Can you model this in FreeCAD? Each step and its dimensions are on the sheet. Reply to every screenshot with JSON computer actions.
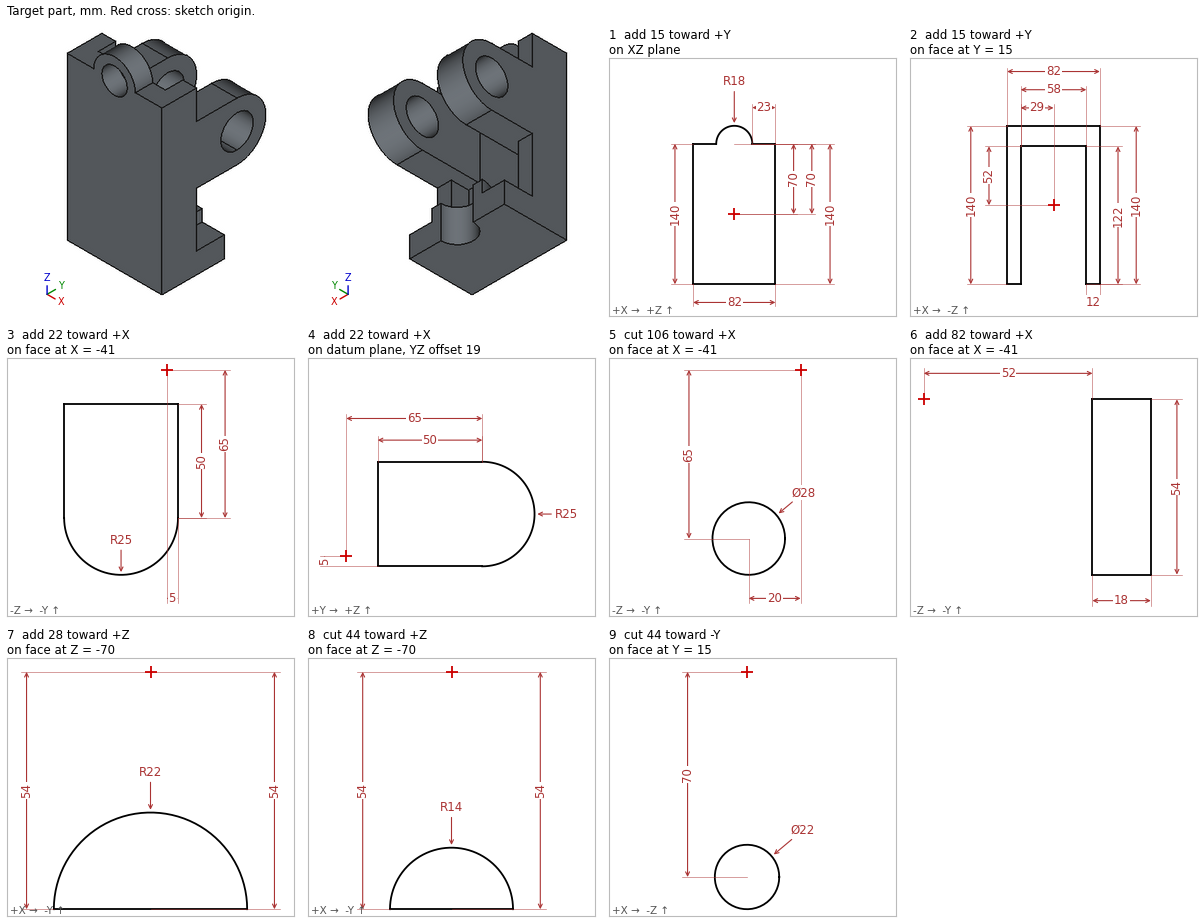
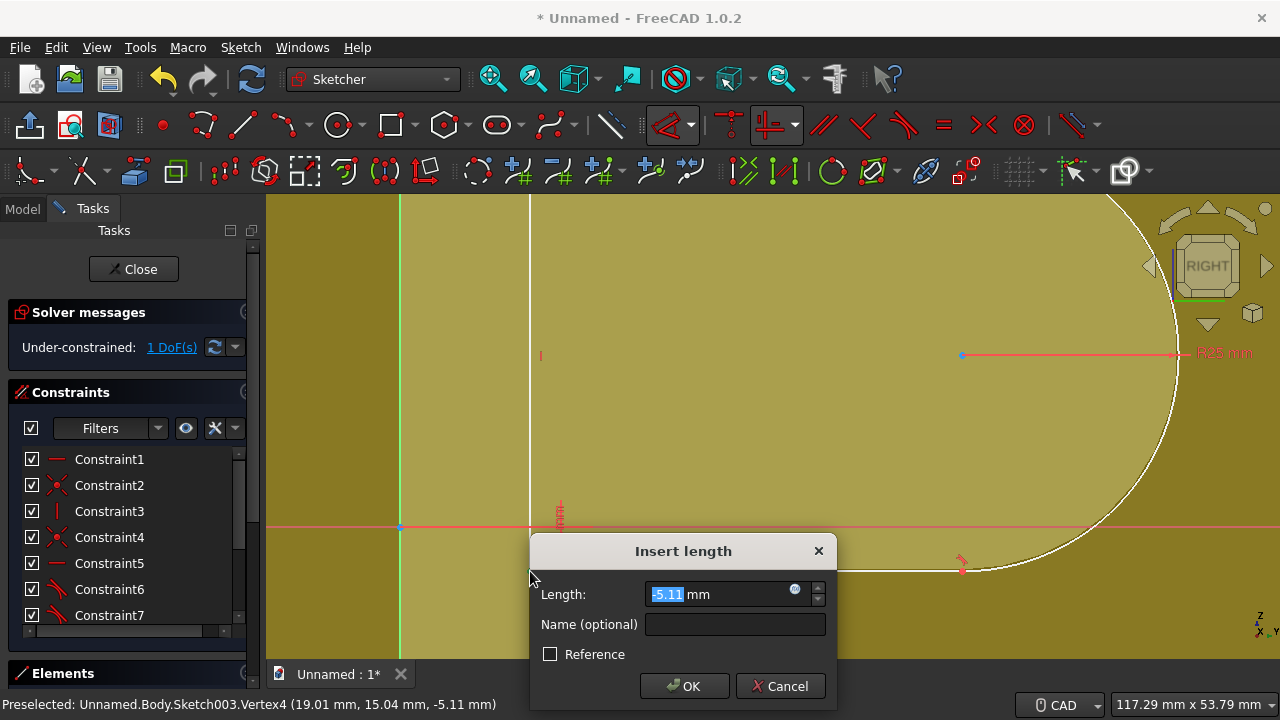
{"action": "type", "text": "-5"}
{"action": "key", "text": "Return"}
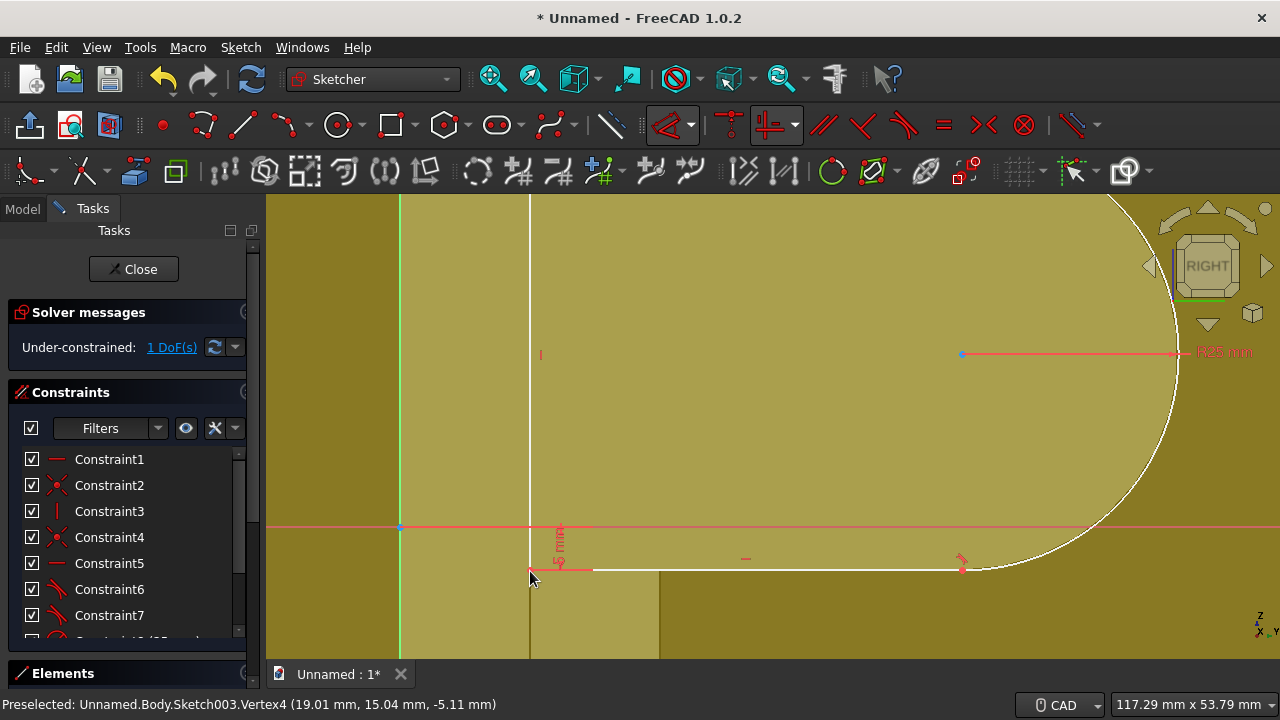
{"action": "scroll", "coordinate": [532, 573], "scroll_direction": "down", "scroll_amount": 2}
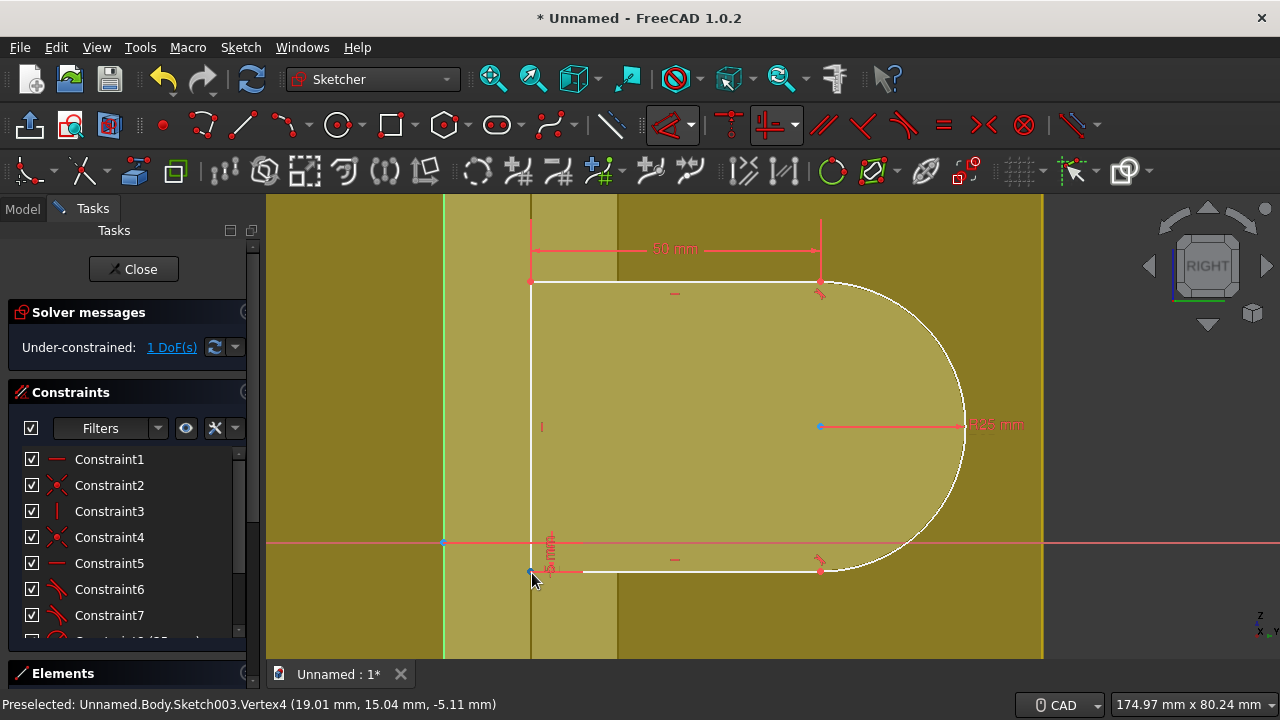
{"action": "left_click", "coordinate": [821, 282]}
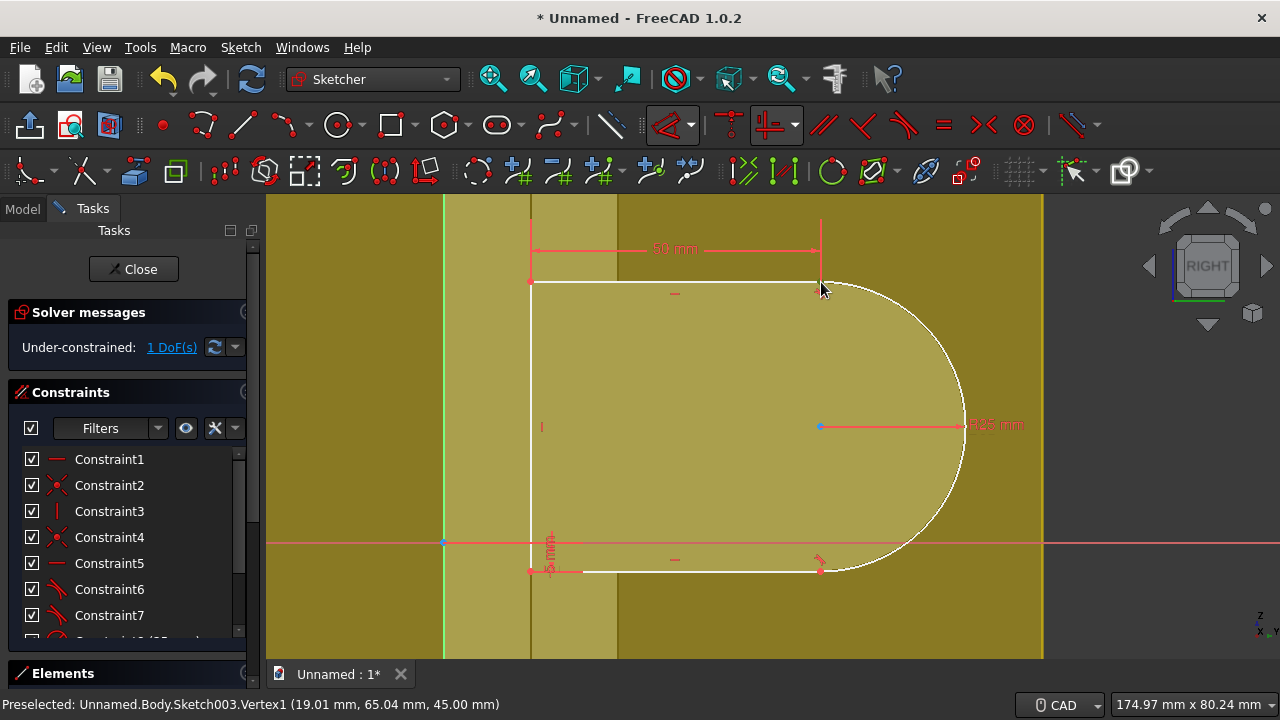
{"action": "key", "text": "l"}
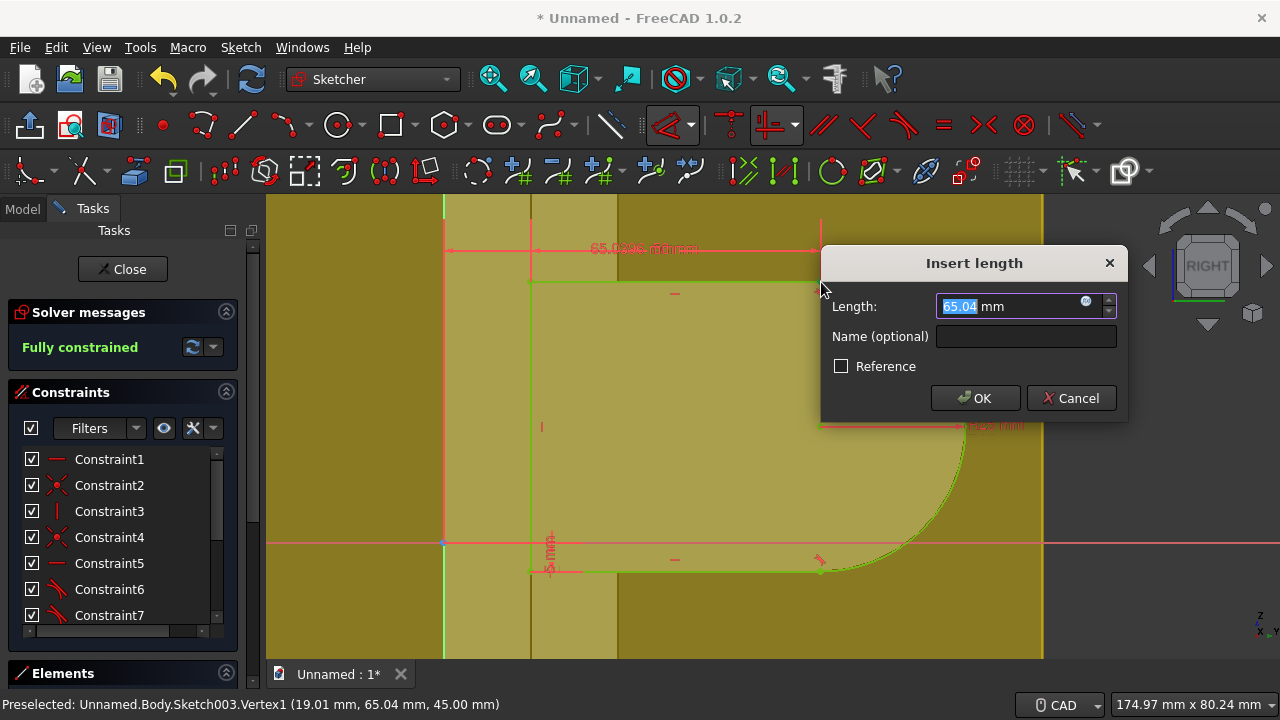
{"action": "type", "text": "65"}
{"action": "key", "text": "Return"}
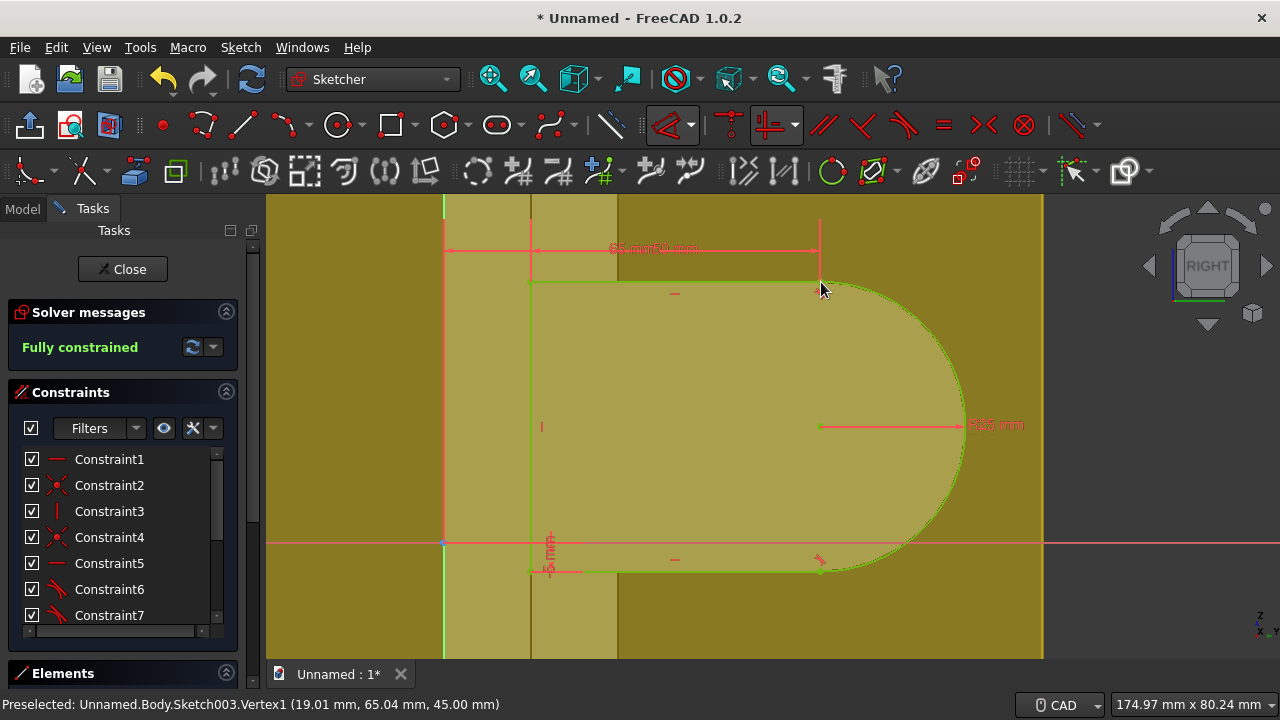
{"action": "left_click", "coordinate": [123, 269]}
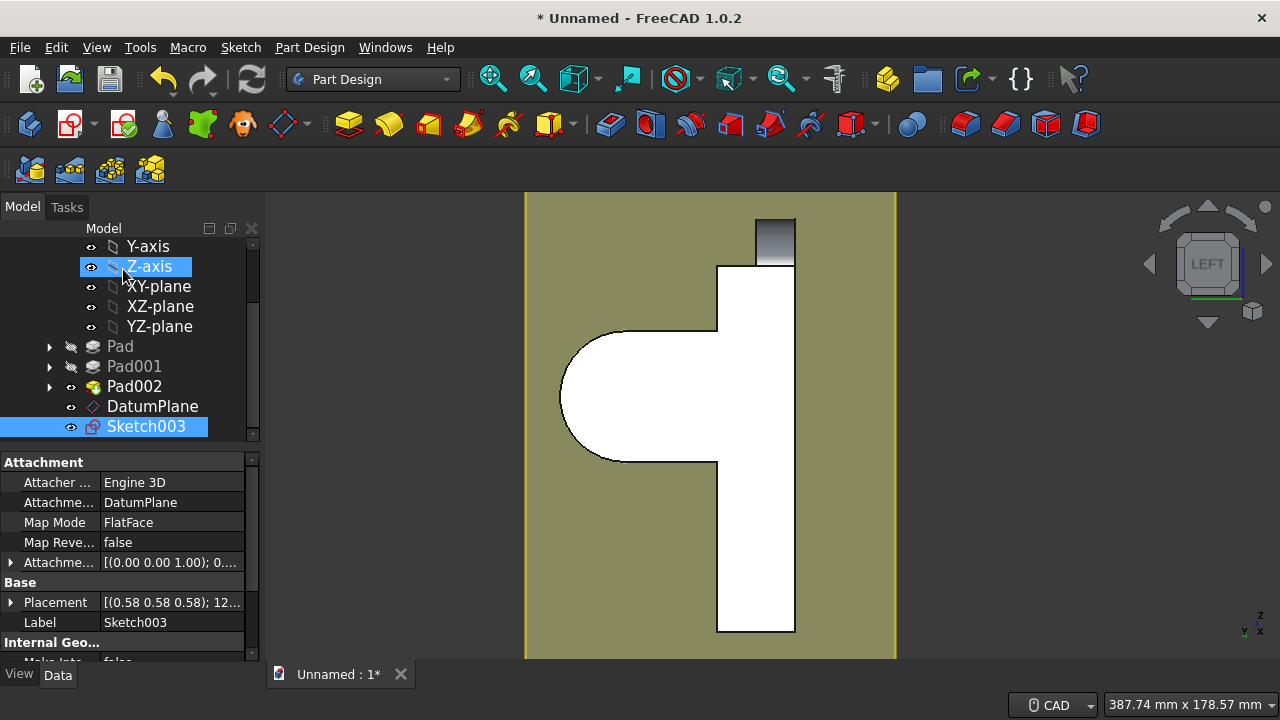
{"action": "left_click", "coordinate": [350, 124]}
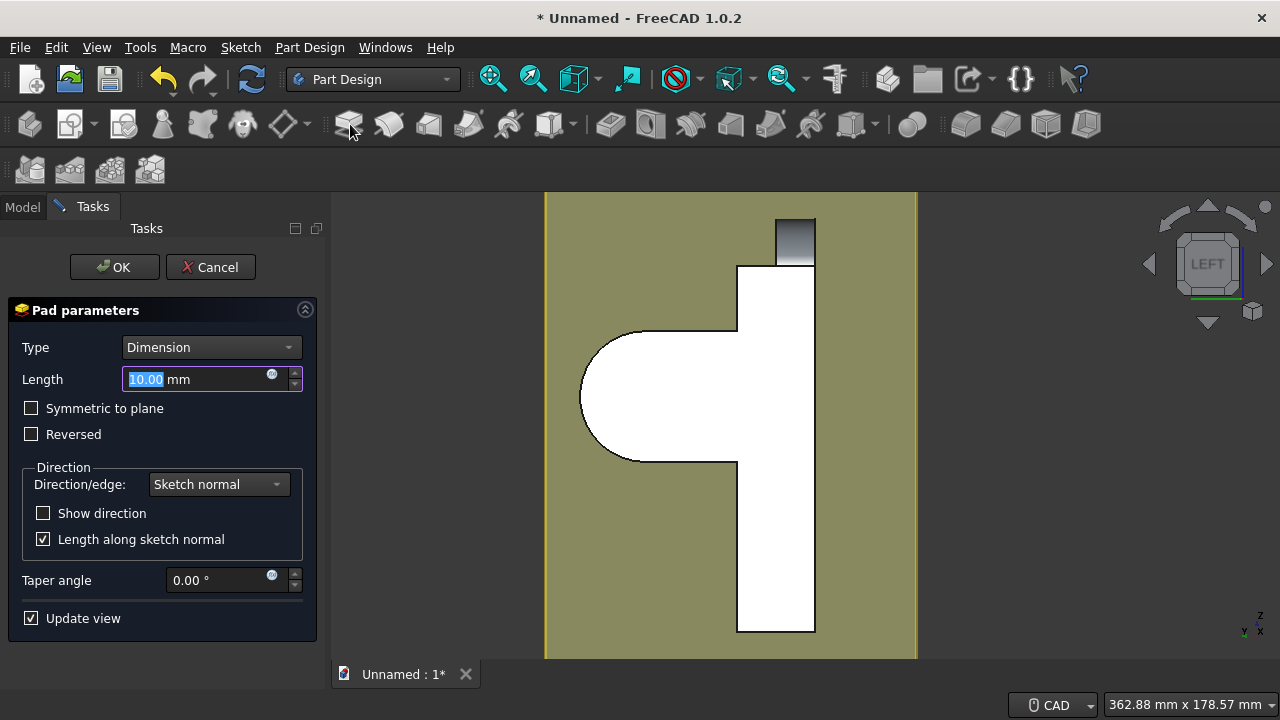
{"action": "type", "text": "22"}
{"action": "key", "text": "Tab"}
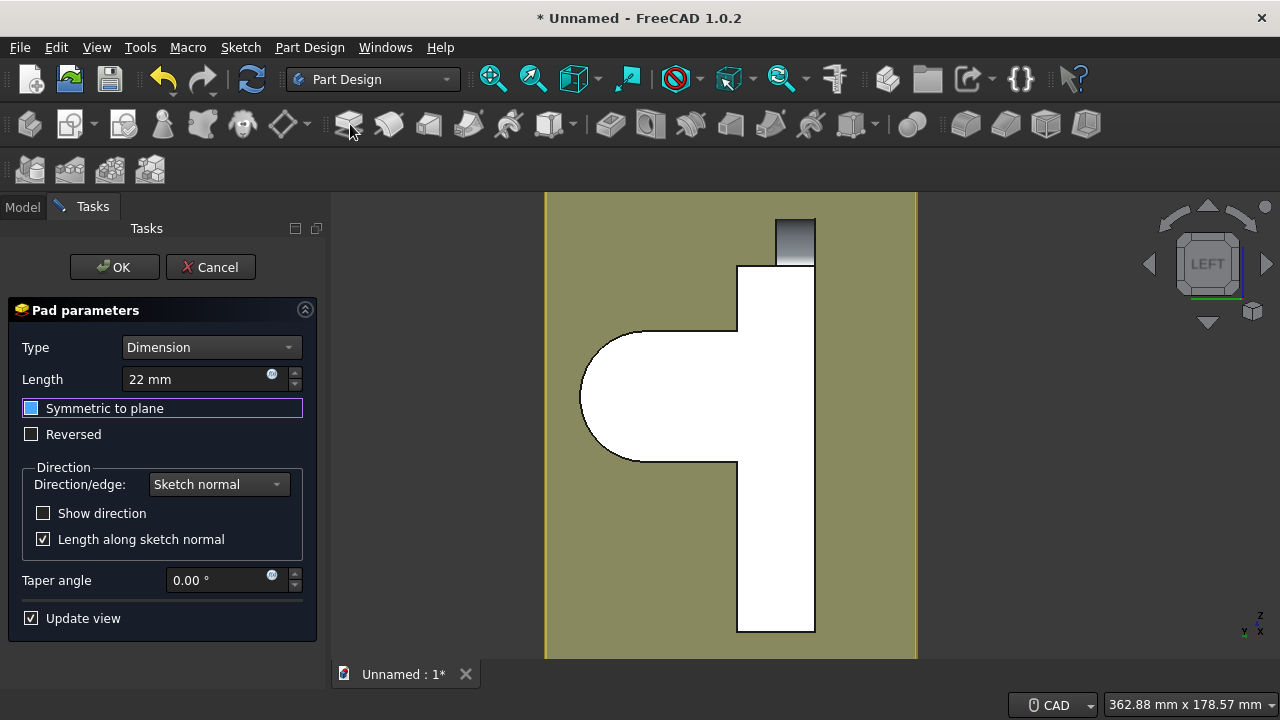
{"action": "left_click", "coordinate": [115, 267]}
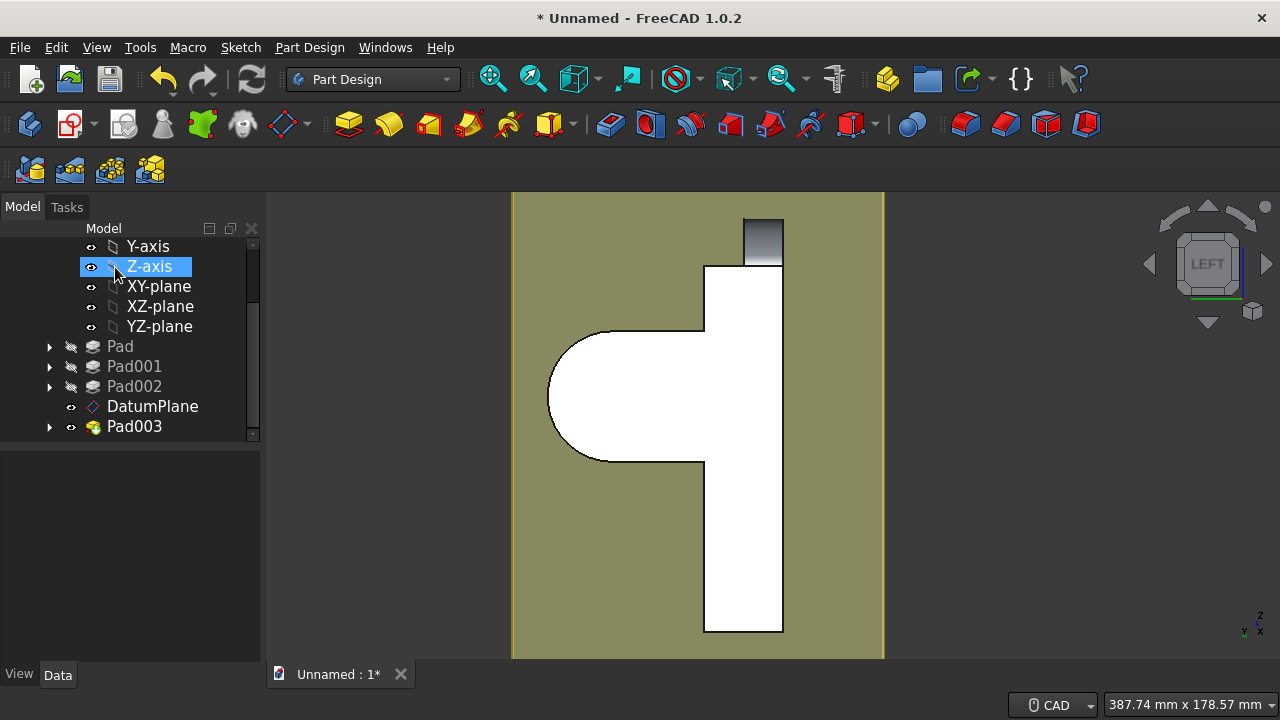
{"action": "left_click", "coordinate": [116, 407]}
{"action": "key", "text": "space"}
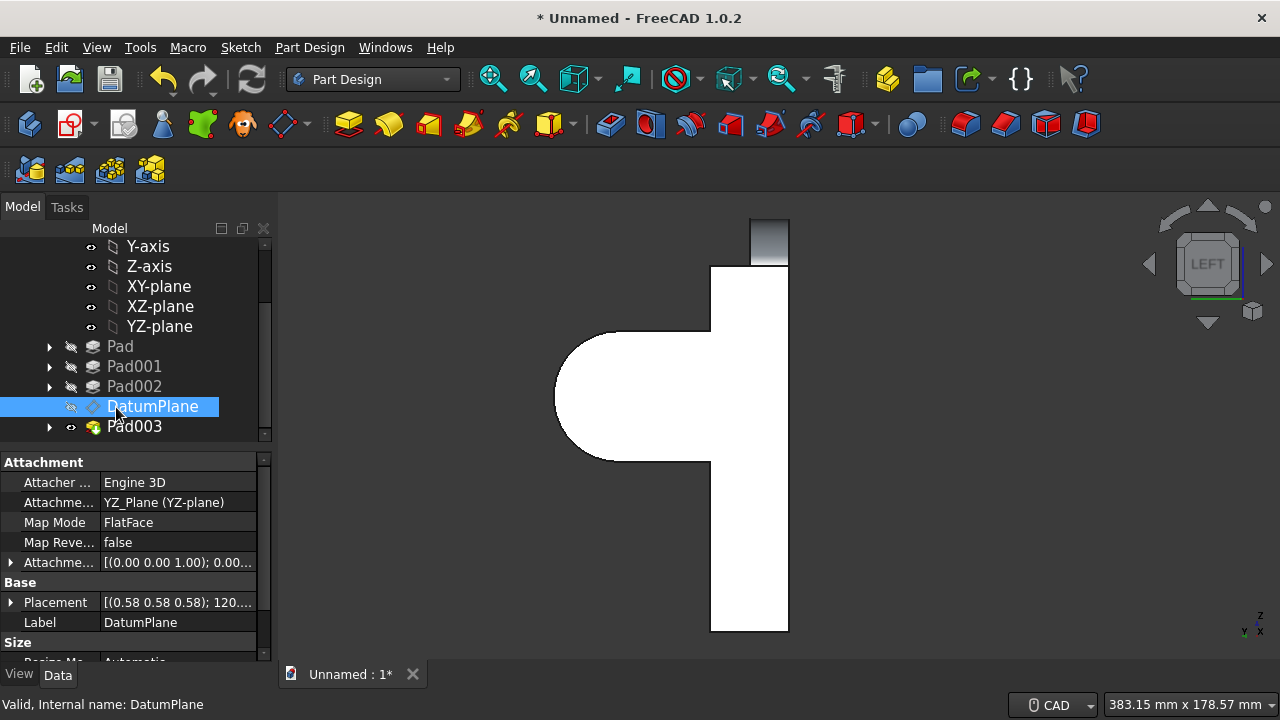
{"action": "left_click", "coordinate": [671, 396]}